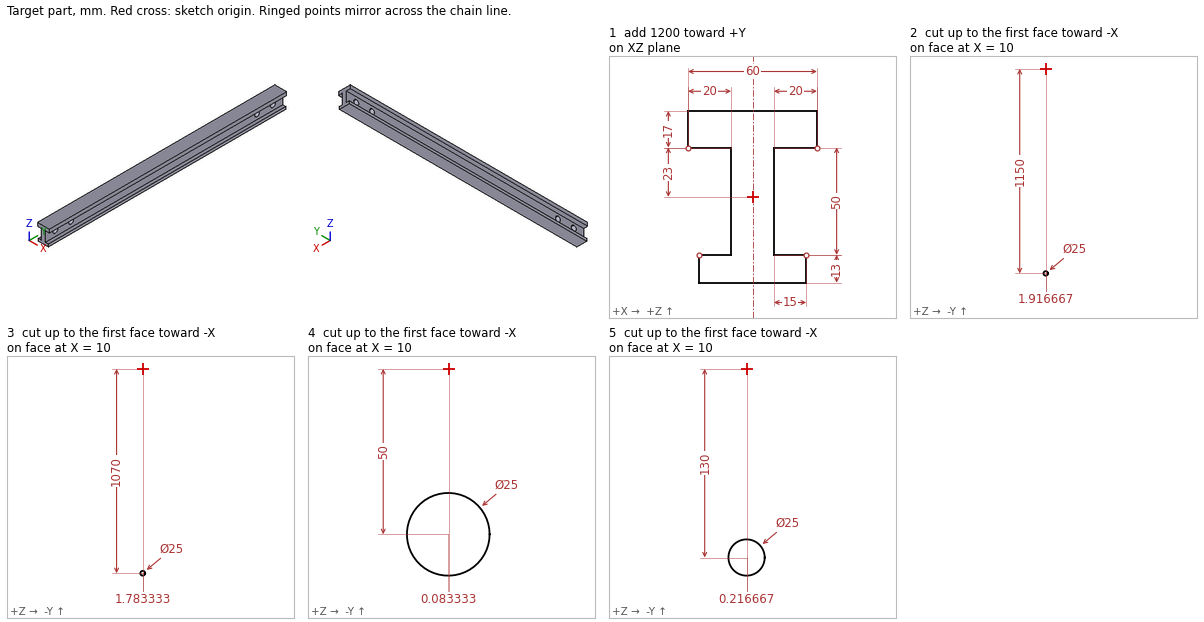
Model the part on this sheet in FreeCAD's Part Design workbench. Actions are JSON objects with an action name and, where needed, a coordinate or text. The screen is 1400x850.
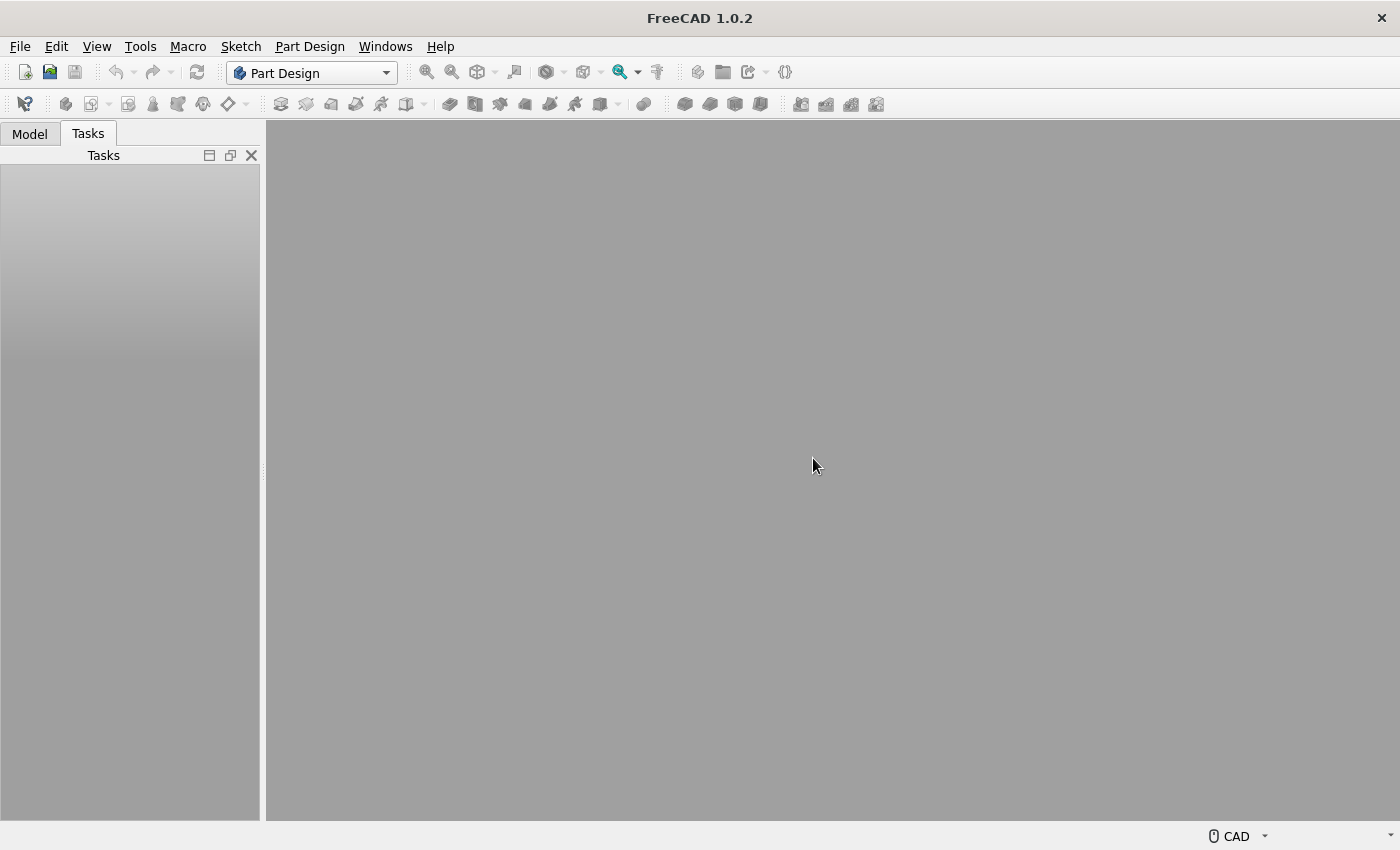
{"action": "left_click", "coordinate": [25, 72]}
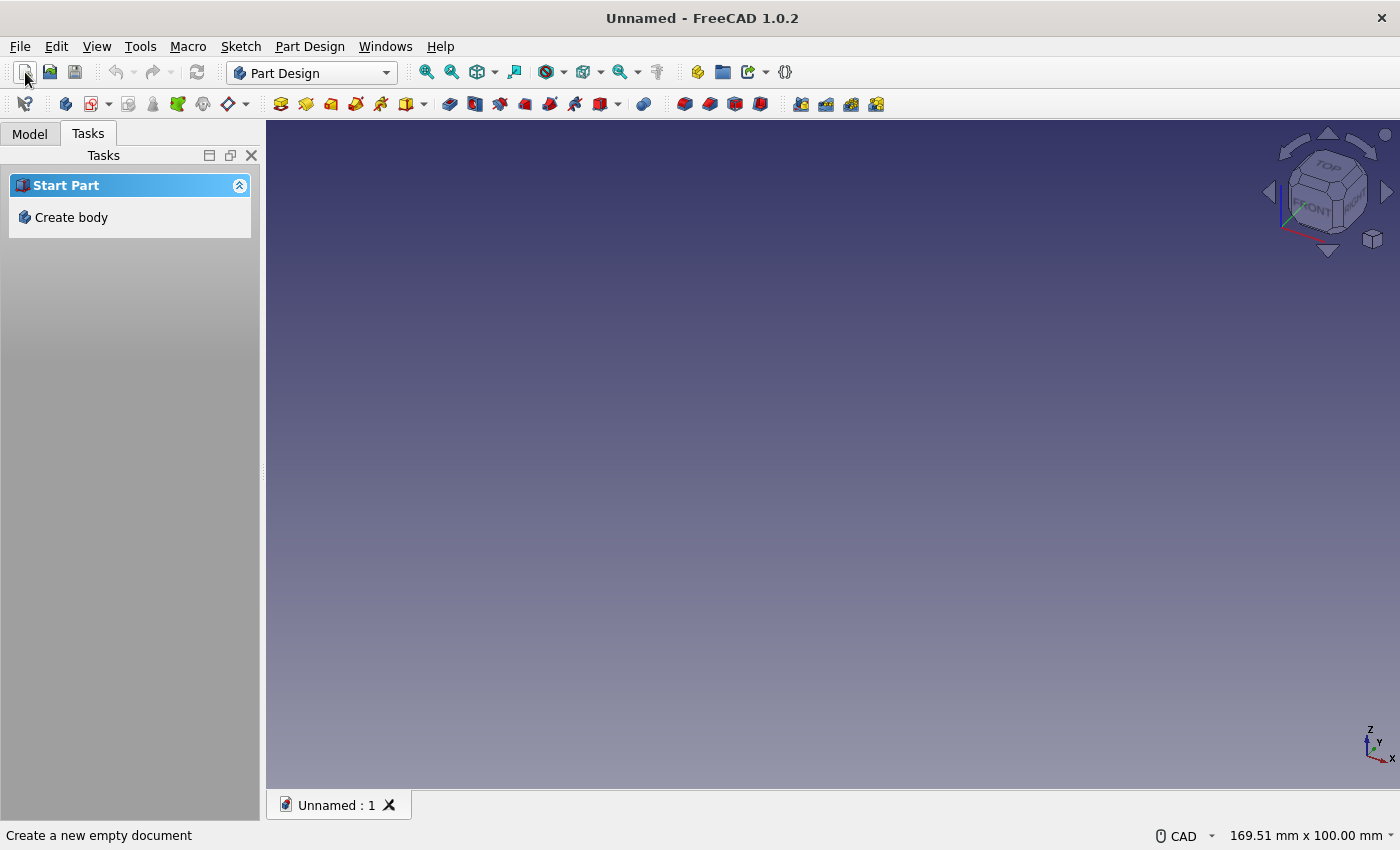
{"action": "left_click", "coordinate": [90, 104]}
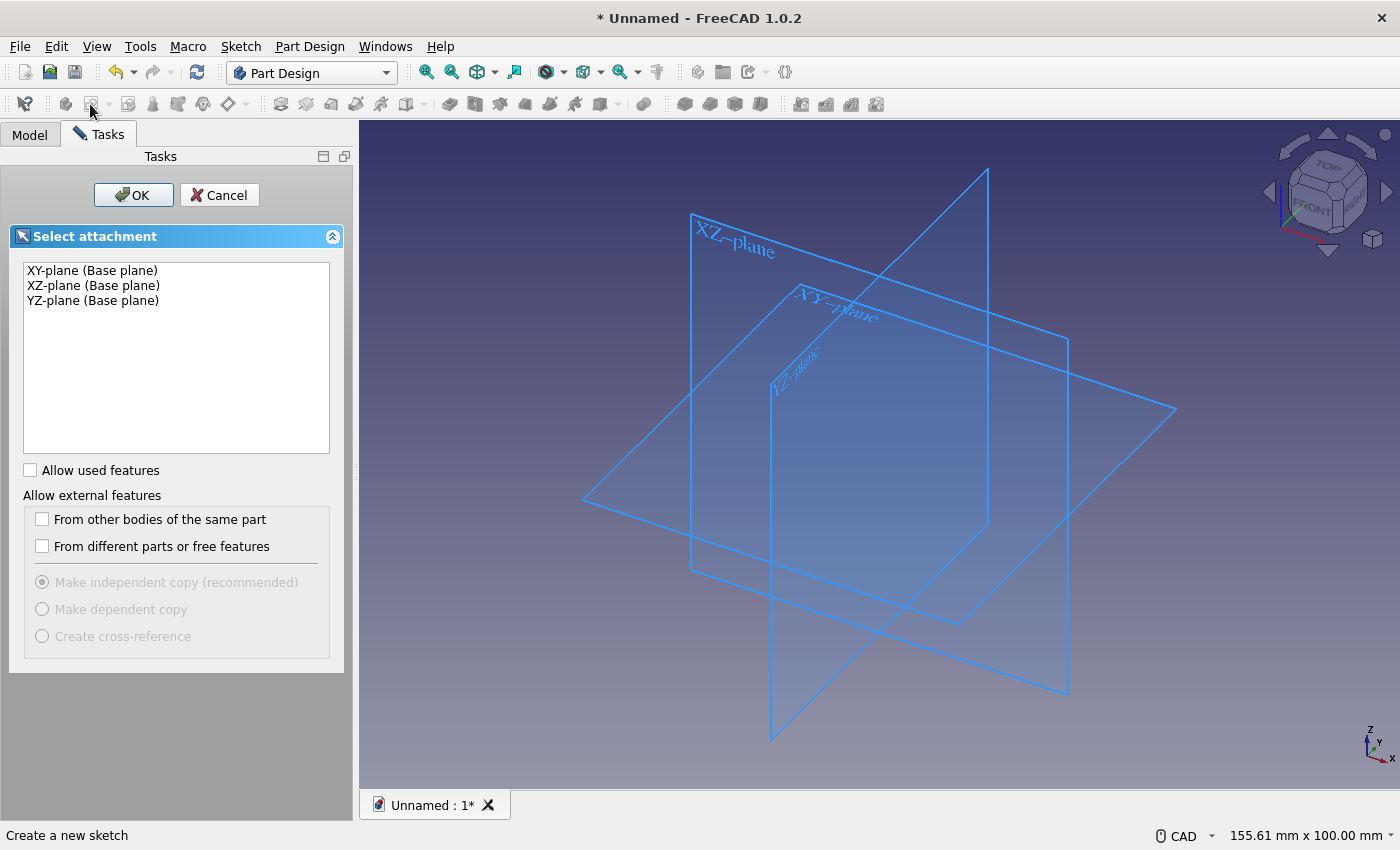
{"action": "left_click", "coordinate": [84, 286]}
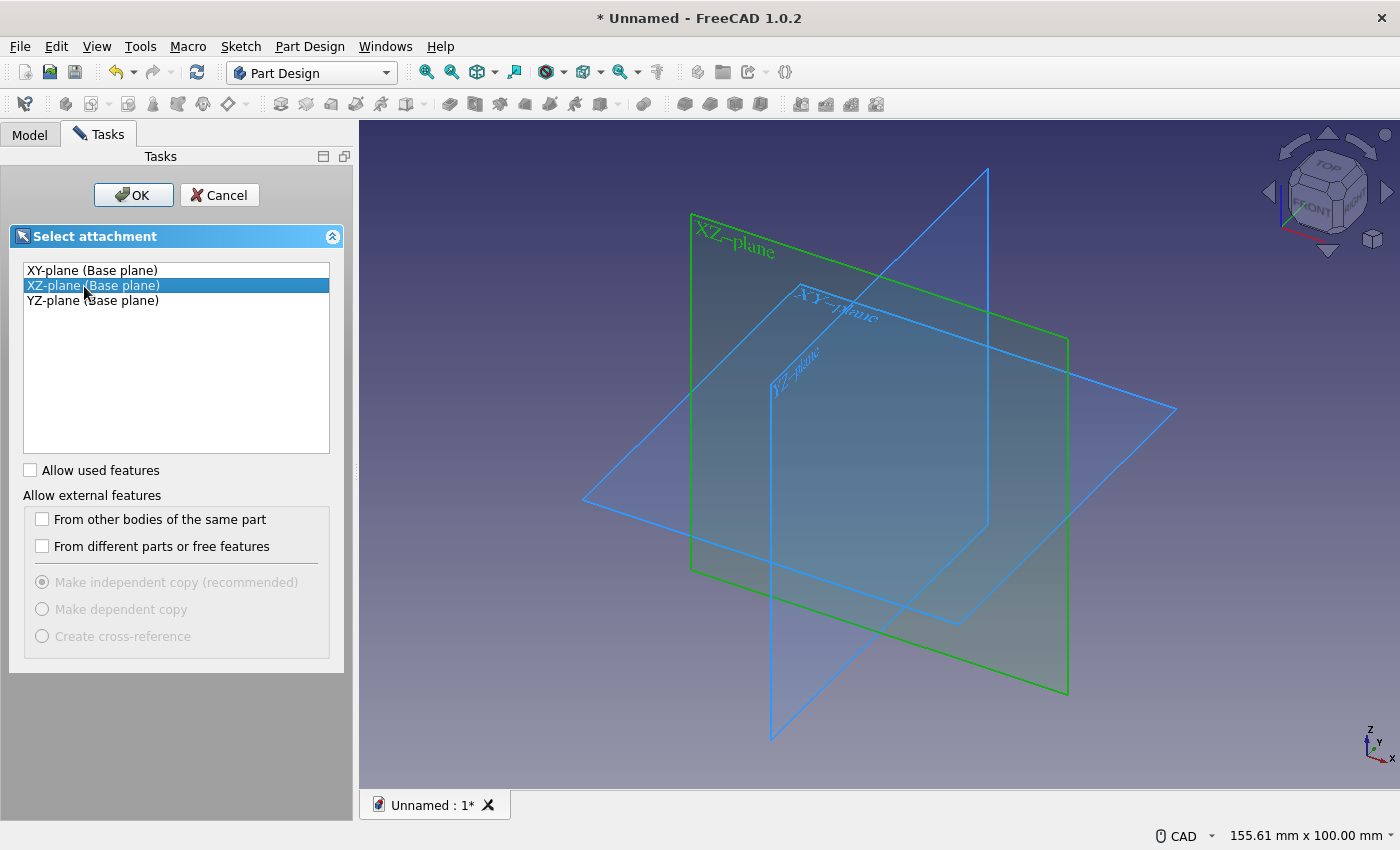
{"action": "left_click", "coordinate": [134, 195]}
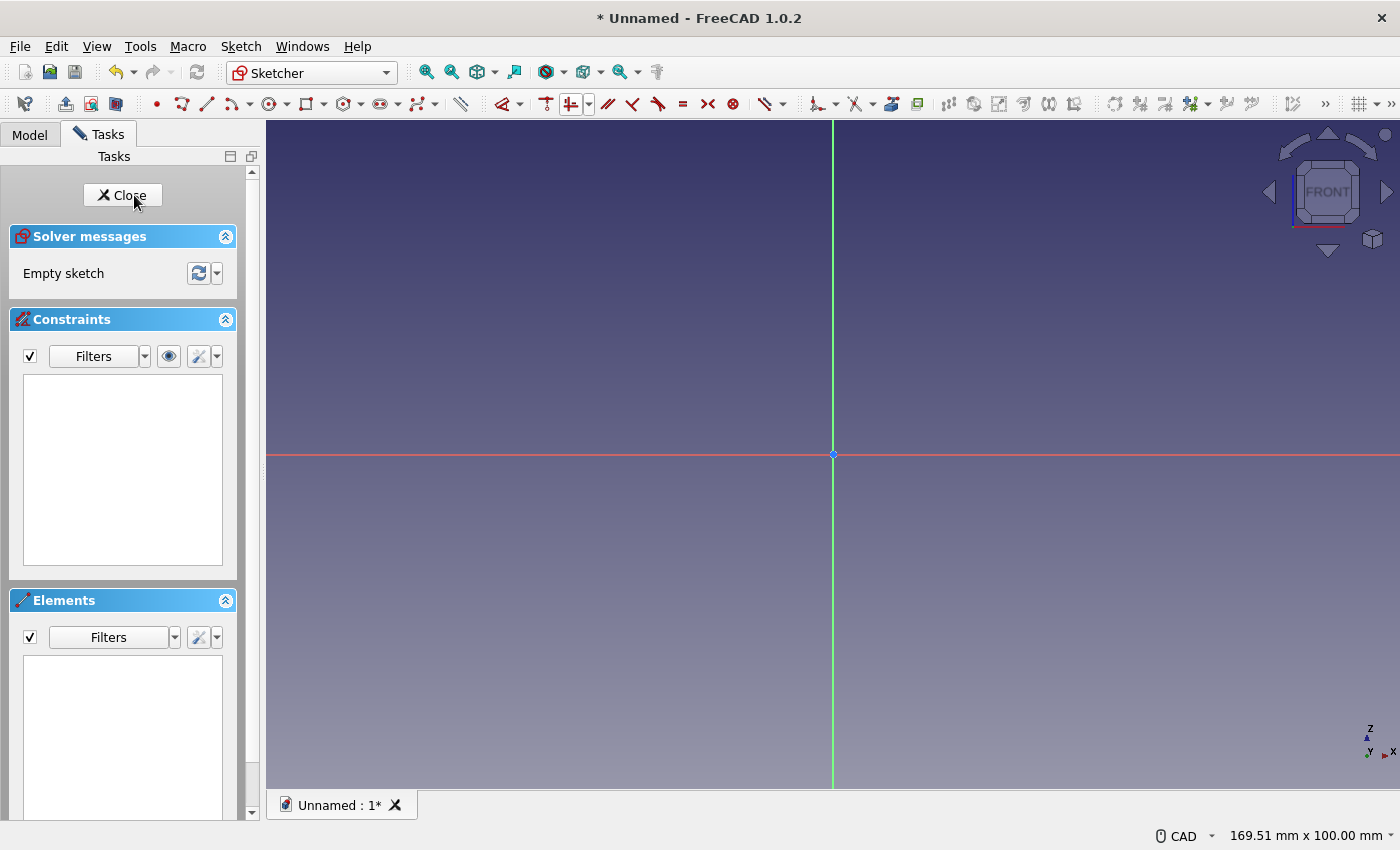
{"action": "left_click", "coordinate": [182, 104]}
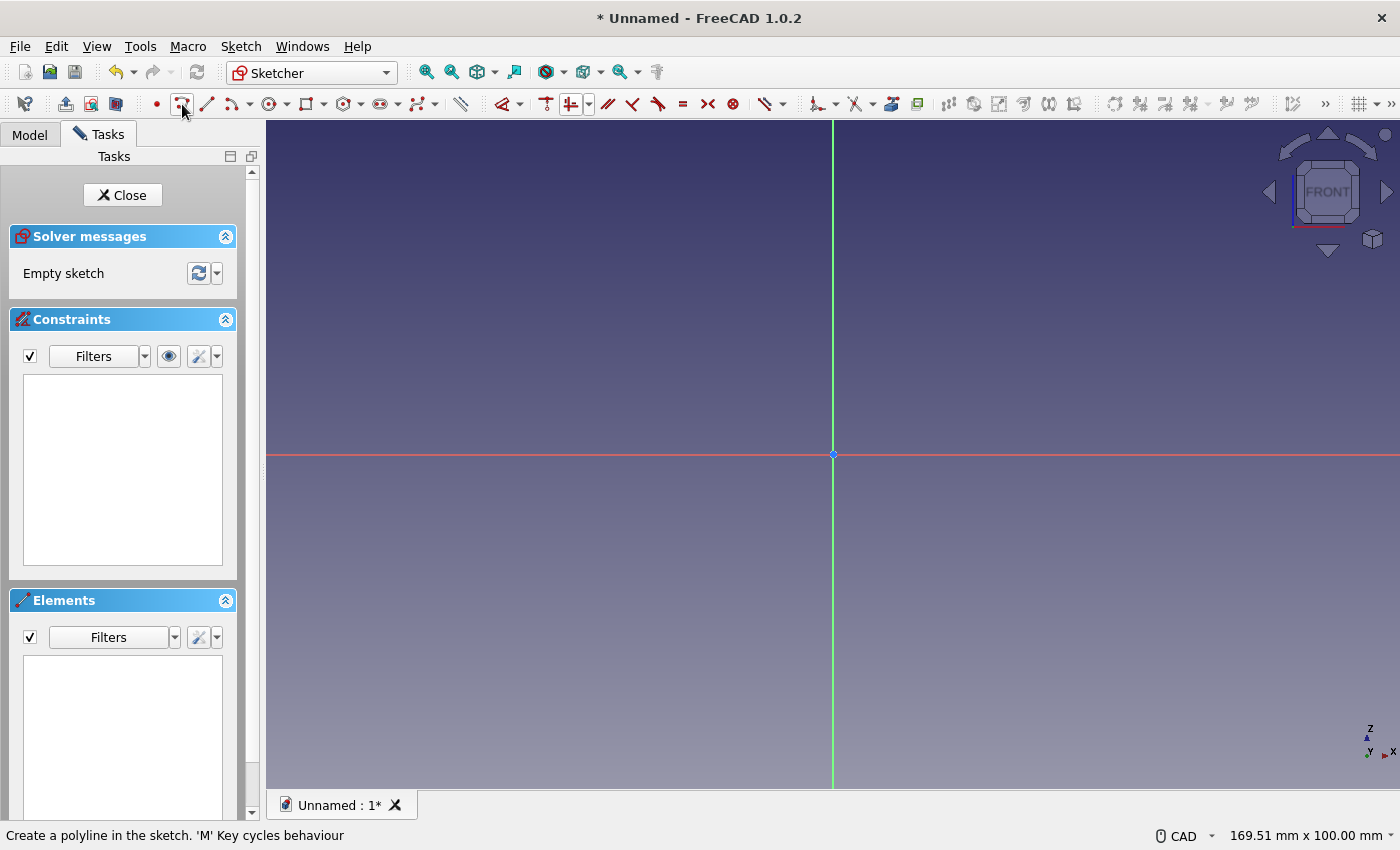
{"action": "left_click", "coordinate": [766, 301]}
{"action": "left_click", "coordinate": [632, 301]}
{"action": "left_click", "coordinate": [632, 187]}
{"action": "left_click", "coordinate": [1034, 187]}
{"action": "left_click", "coordinate": [1034, 301]}
{"action": "left_click", "coordinate": [900, 301]}
{"action": "left_click", "coordinate": [900, 635]}
{"action": "left_click", "coordinate": [1000, 635]}
{"action": "left_click", "coordinate": [1000, 722]}
{"action": "left_click", "coordinate": [666, 722]}
{"action": "left_click", "coordinate": [666, 635]}
{"action": "left_click", "coordinate": [766, 635]}
{"action": "left_click", "coordinate": [766, 302]}
{"action": "key", "text": "Escape"}
{"action": "key", "text": "Escape"}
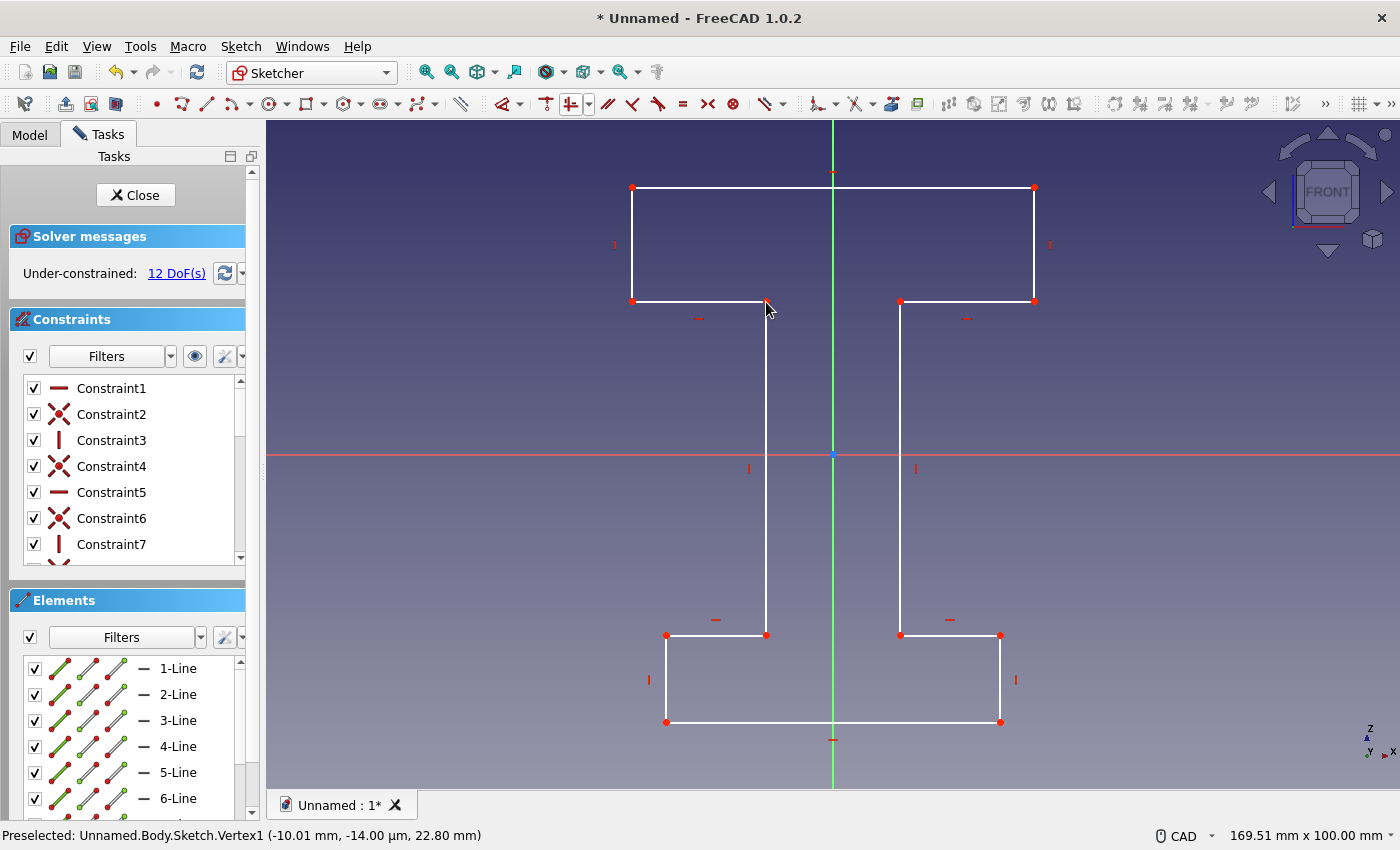
{"action": "left_click", "coordinate": [632, 302]}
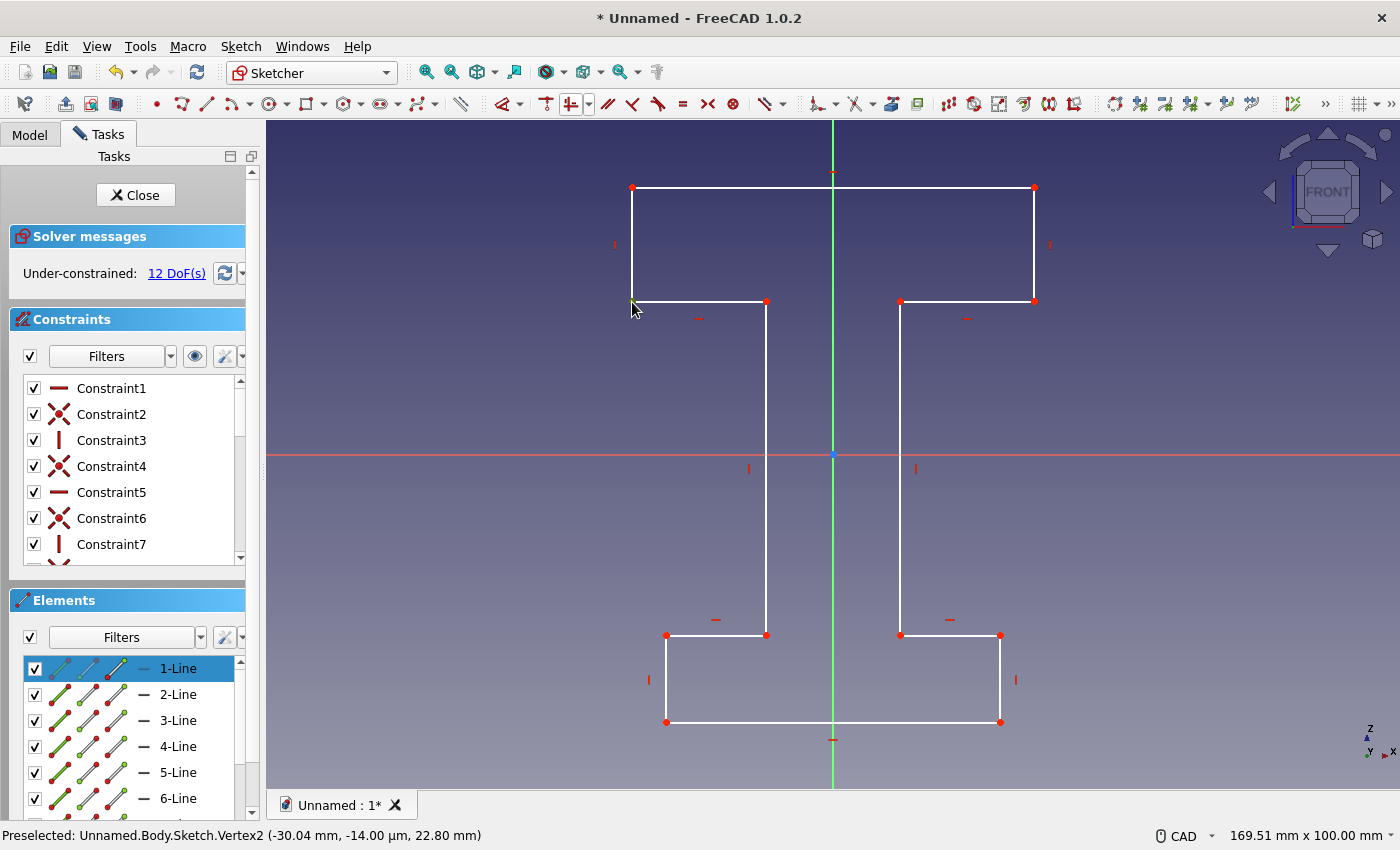
{"action": "left_click", "coordinate": [1034, 302]}